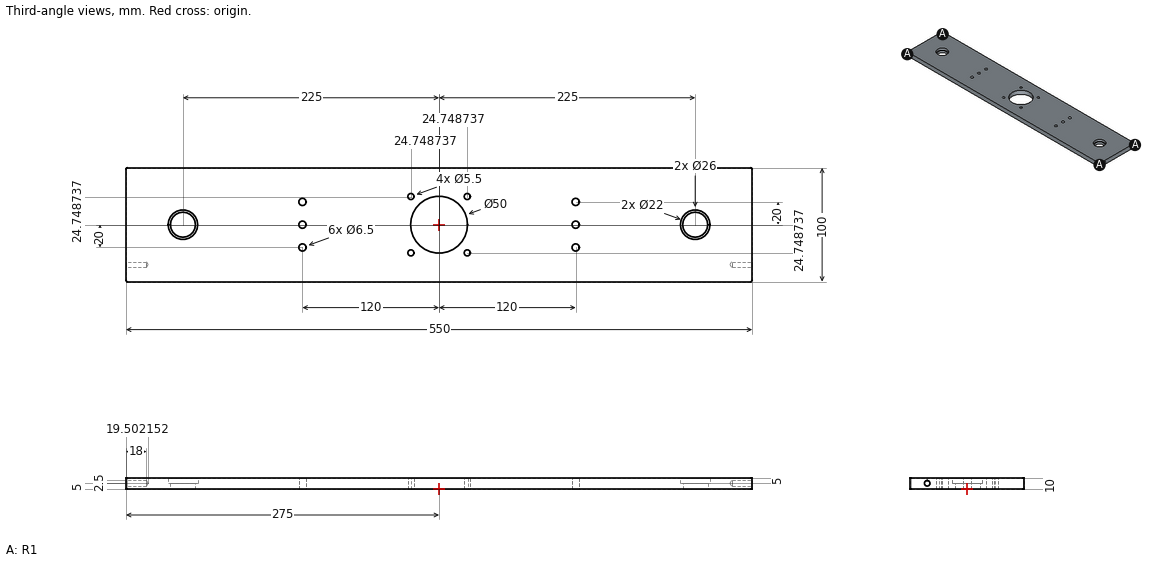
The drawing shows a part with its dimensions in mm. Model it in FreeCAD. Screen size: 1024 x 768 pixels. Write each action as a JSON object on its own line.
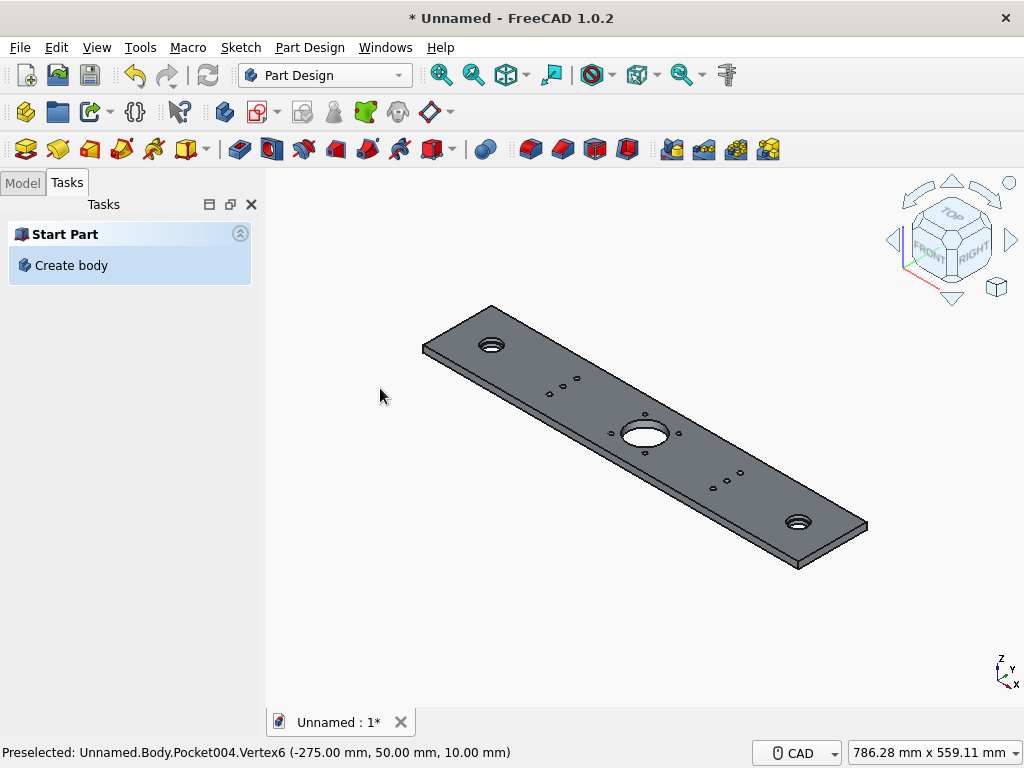
{"action": "left_click", "coordinate": [798, 567]}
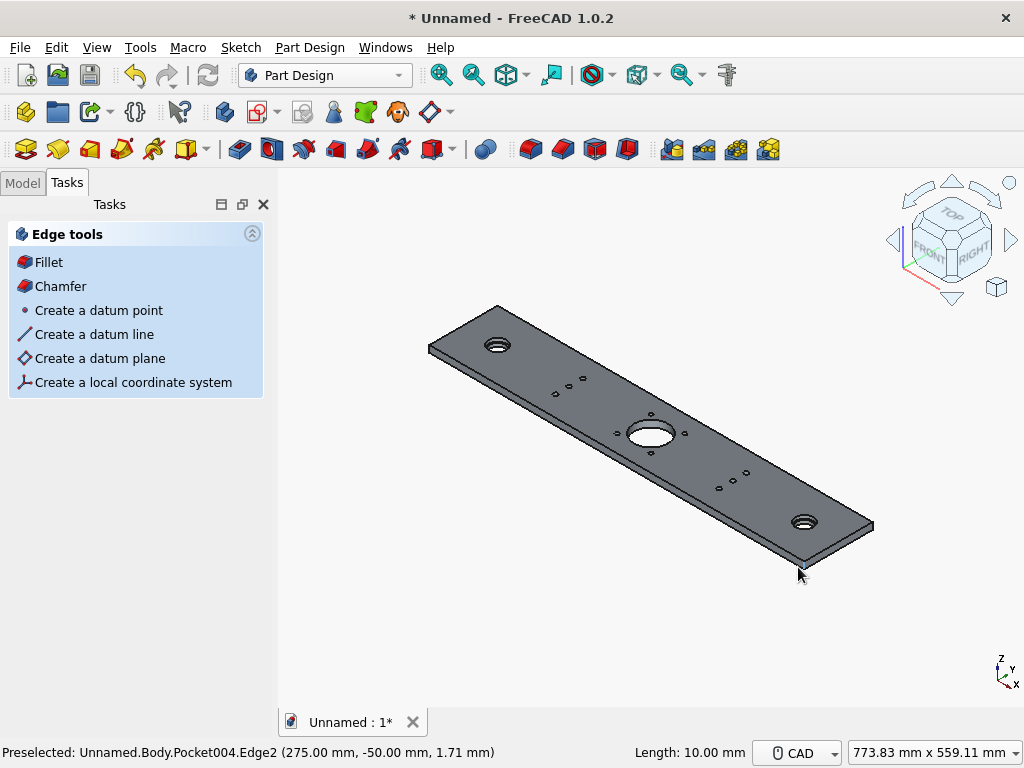
{"action": "scroll", "coordinate": [498, 309], "scroll_direction": "up", "scroll_amount": 8}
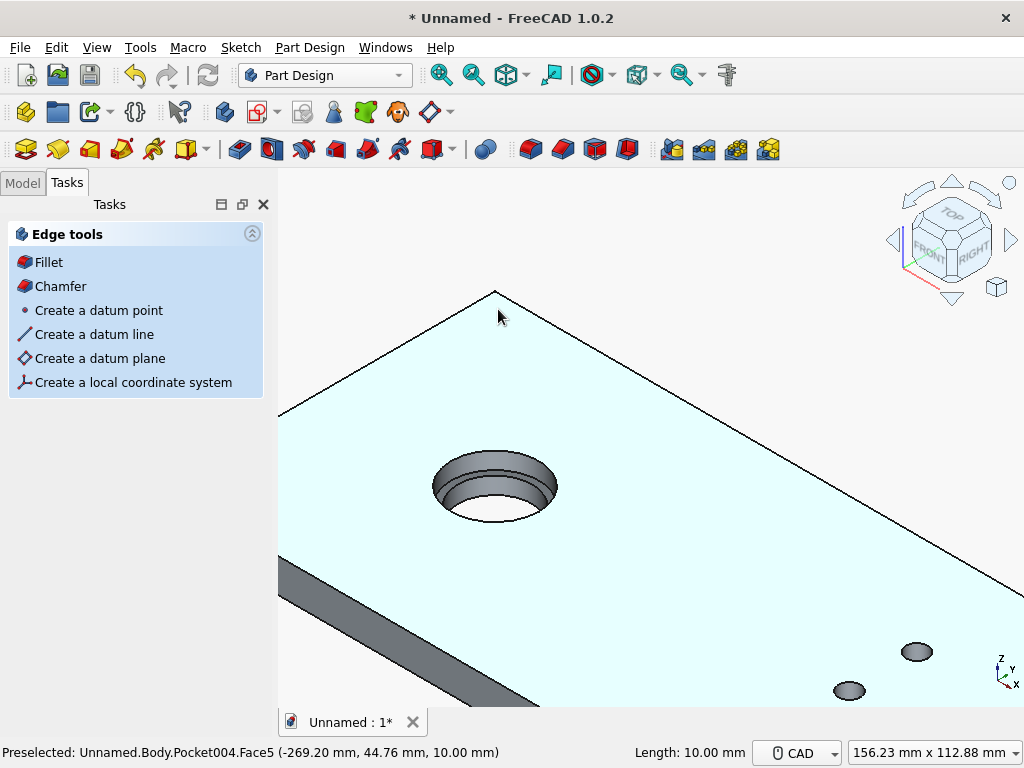
{"action": "left_click", "coordinate": [442, 76]}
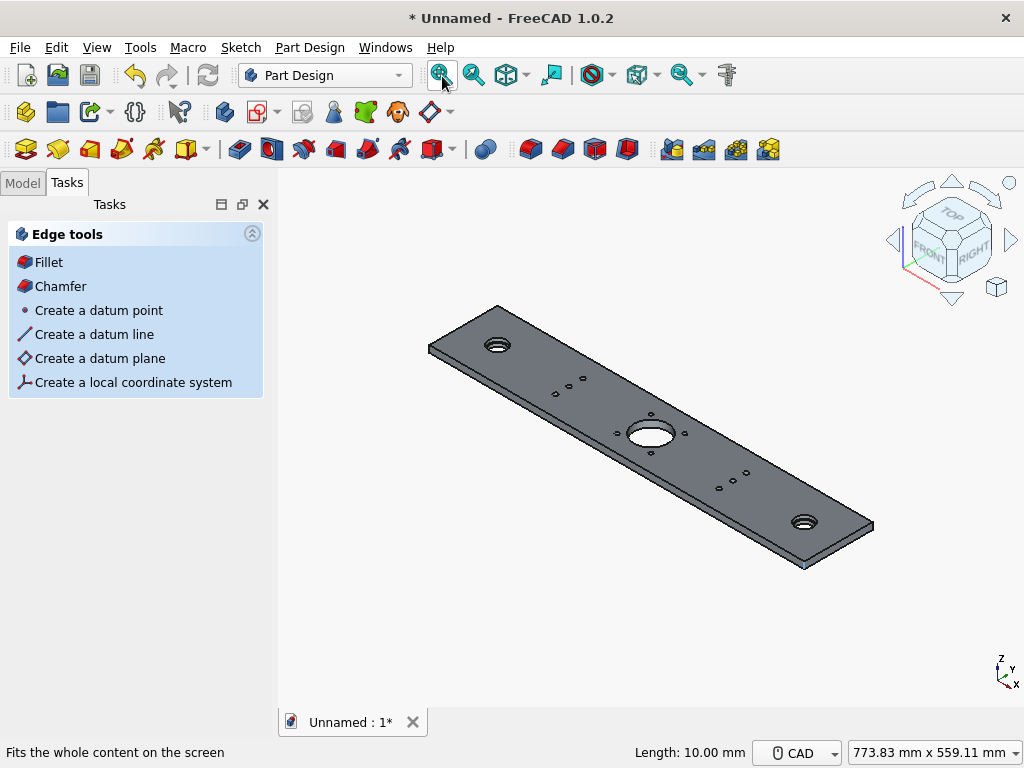
{"action": "key", "text": "2"}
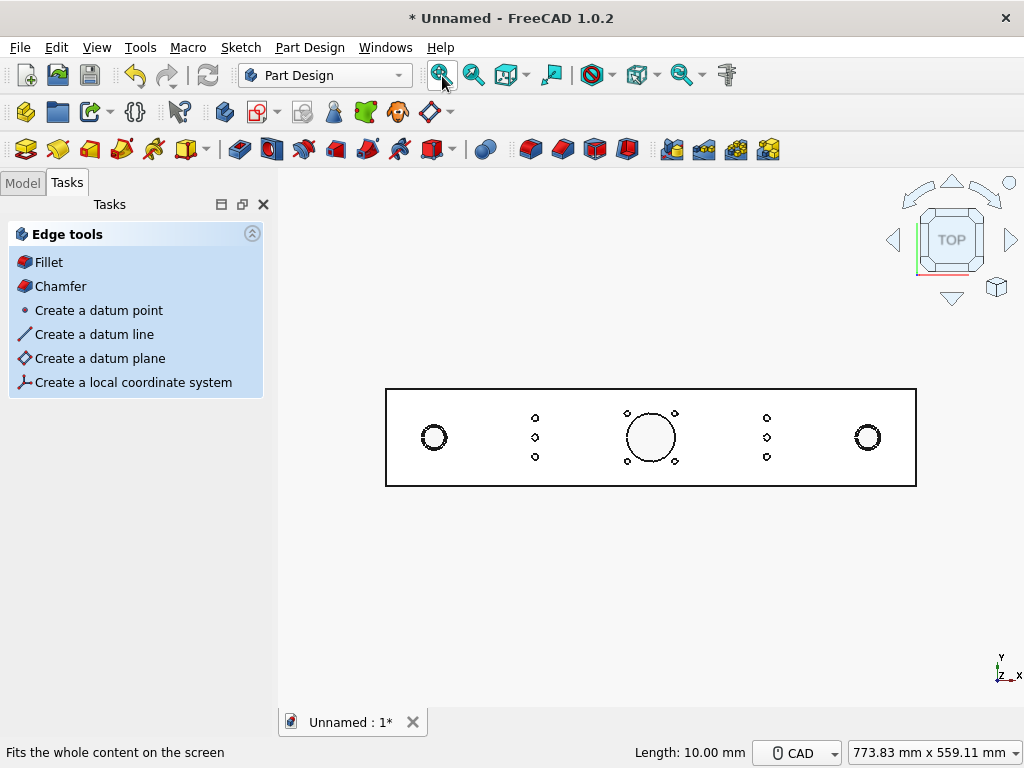
{"action": "scroll", "coordinate": [386, 388], "scroll_direction": "up", "scroll_amount": 8}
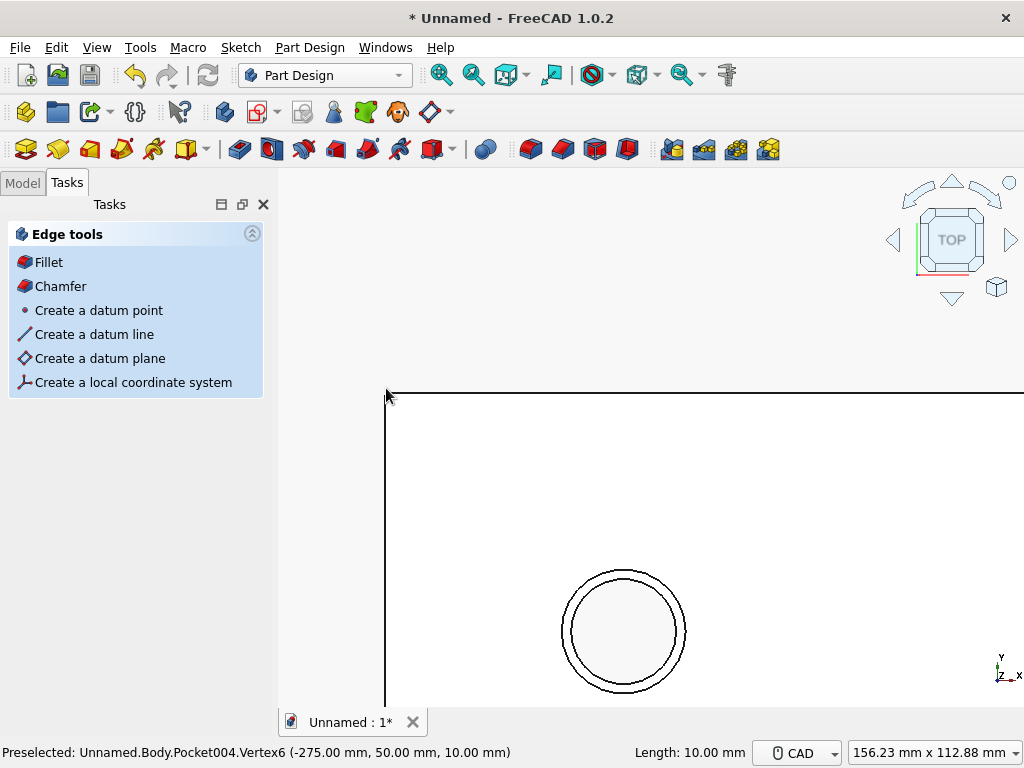
{"action": "key", "text": "v f"}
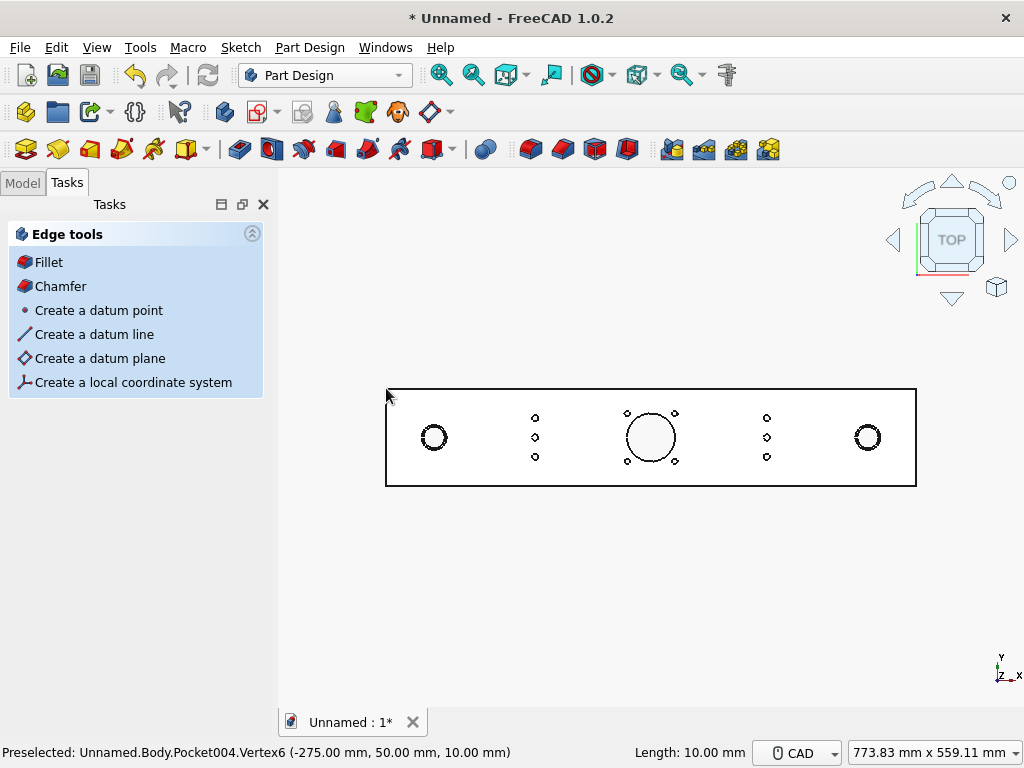
{"action": "key", "text": "1"}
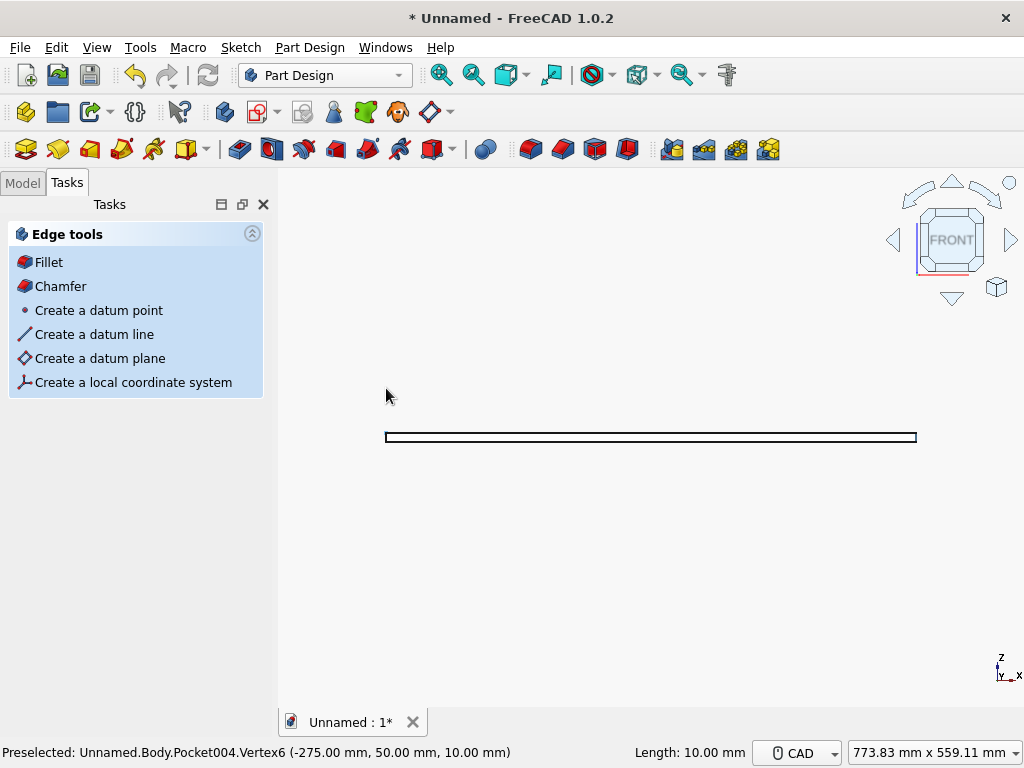
{"action": "scroll", "coordinate": [386, 436], "scroll_direction": "up", "scroll_amount": 8}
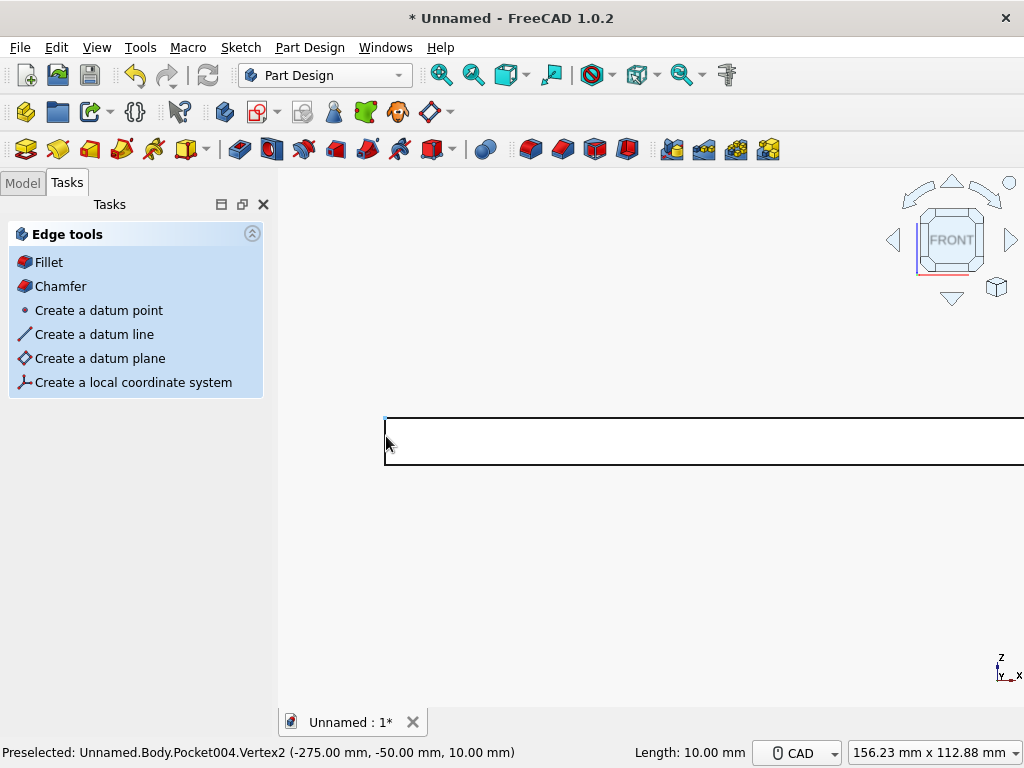
{"action": "left_click", "coordinate": [385, 440], "text": "ctrl"}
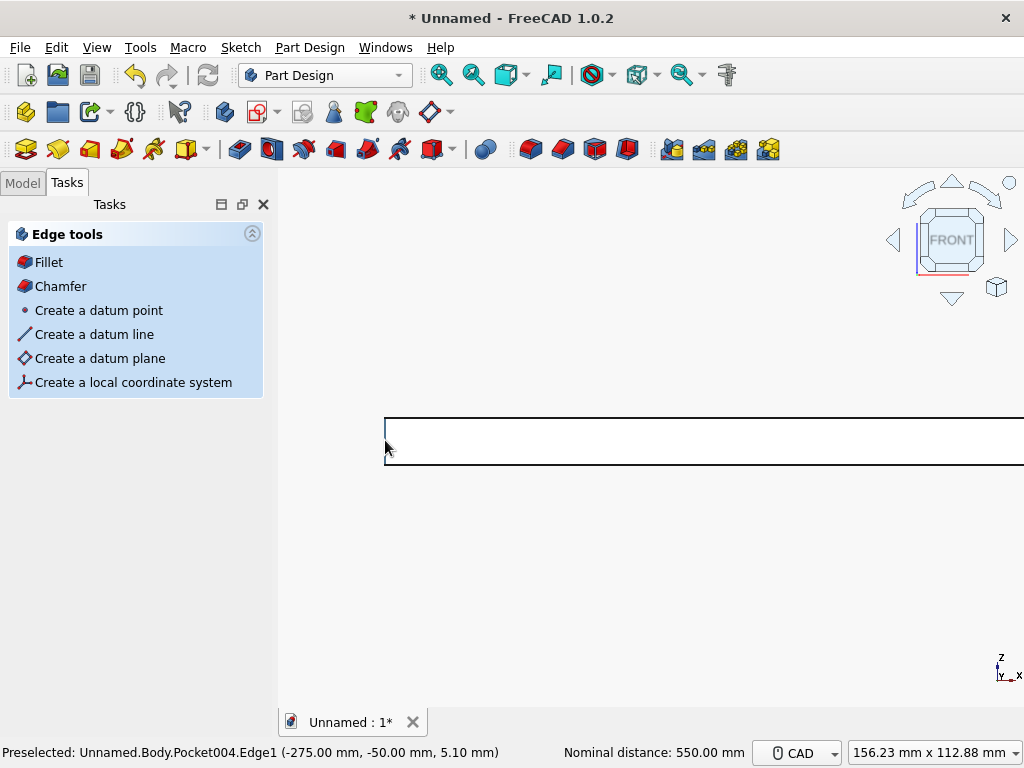
{"action": "left_click", "coordinate": [442, 76]}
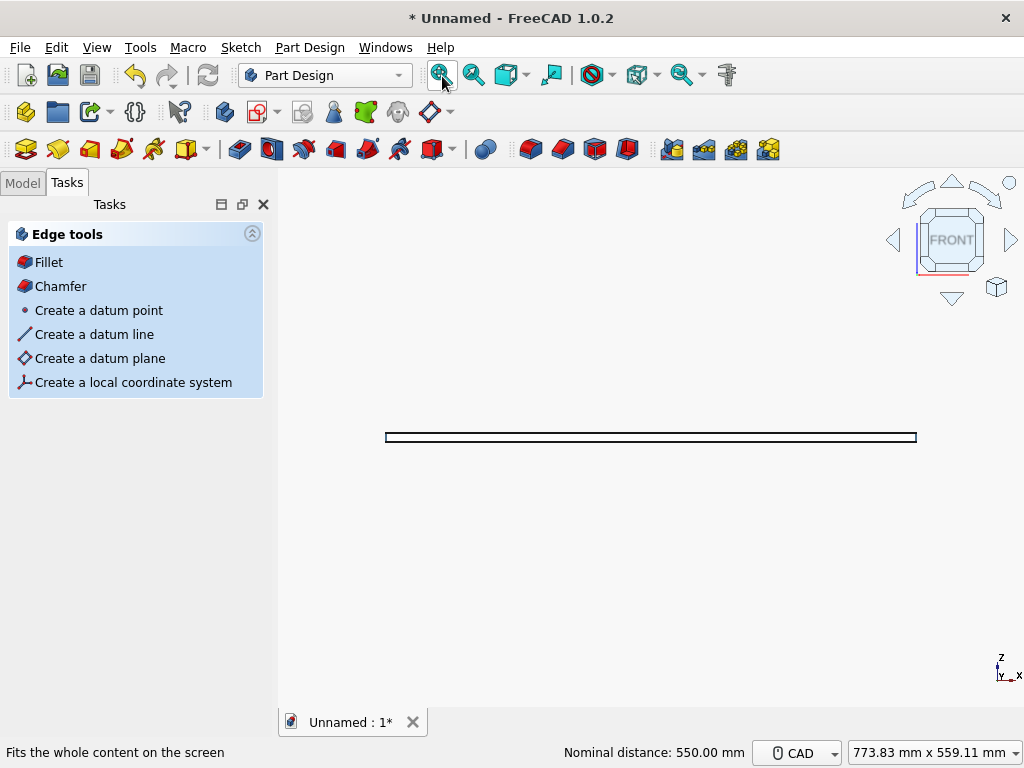
{"action": "key", "text": "3"}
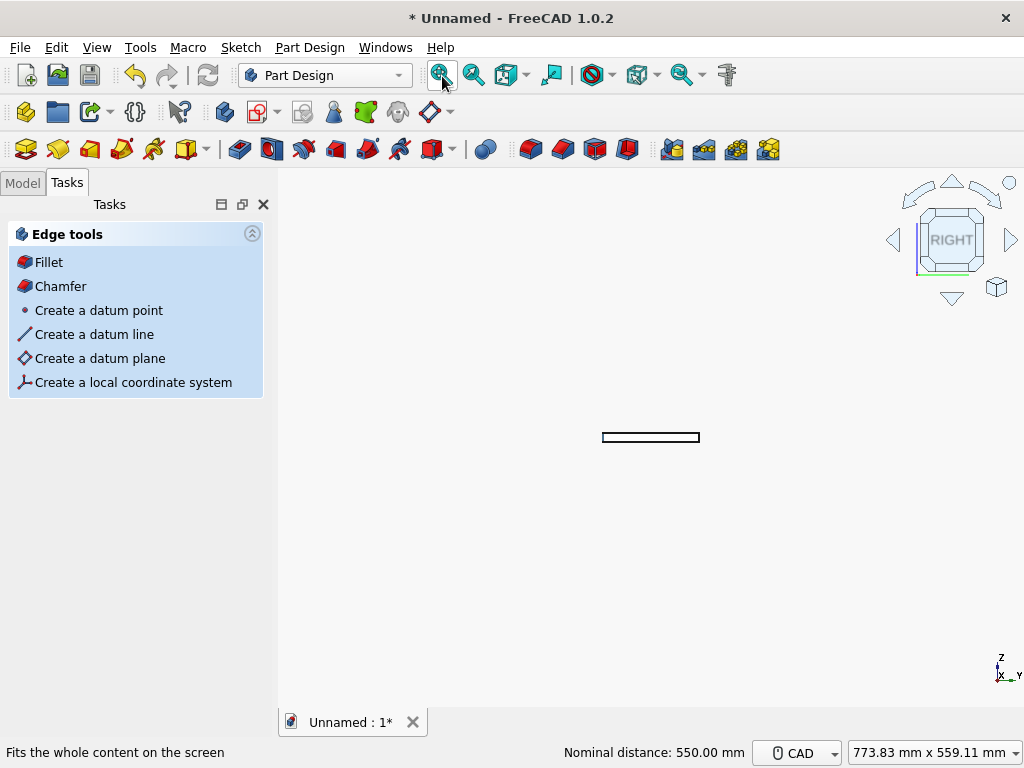
{"action": "left_click", "coordinate": [442, 76]}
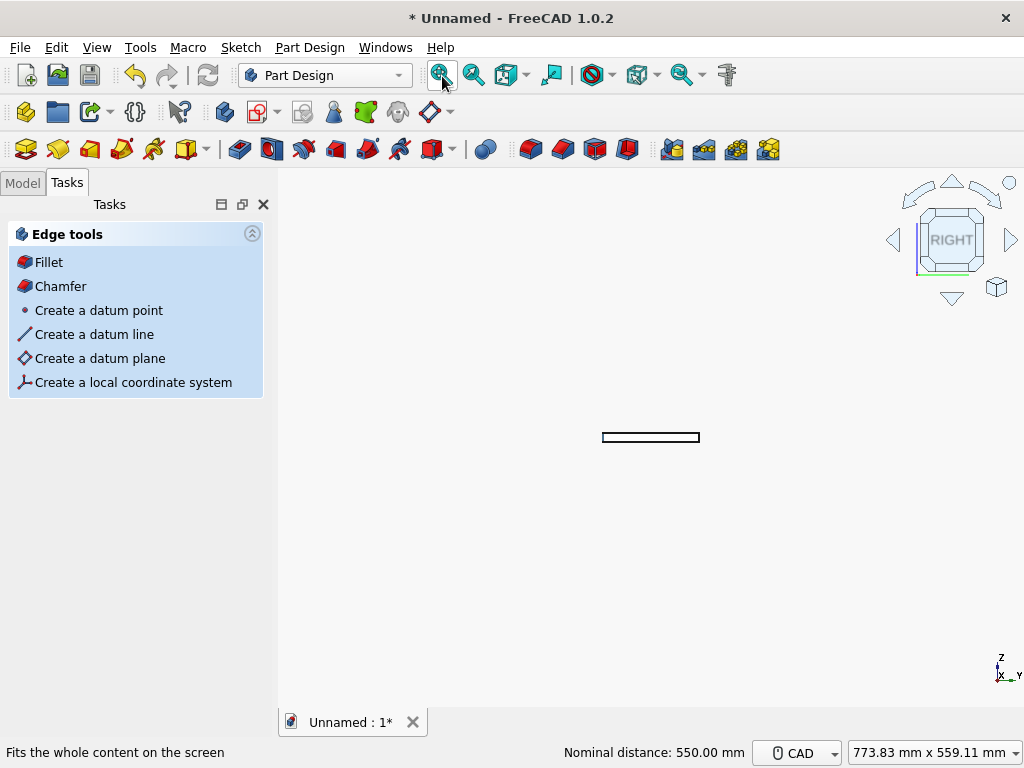
{"action": "scroll", "coordinate": [699, 436], "scroll_direction": "up", "scroll_amount": 8}